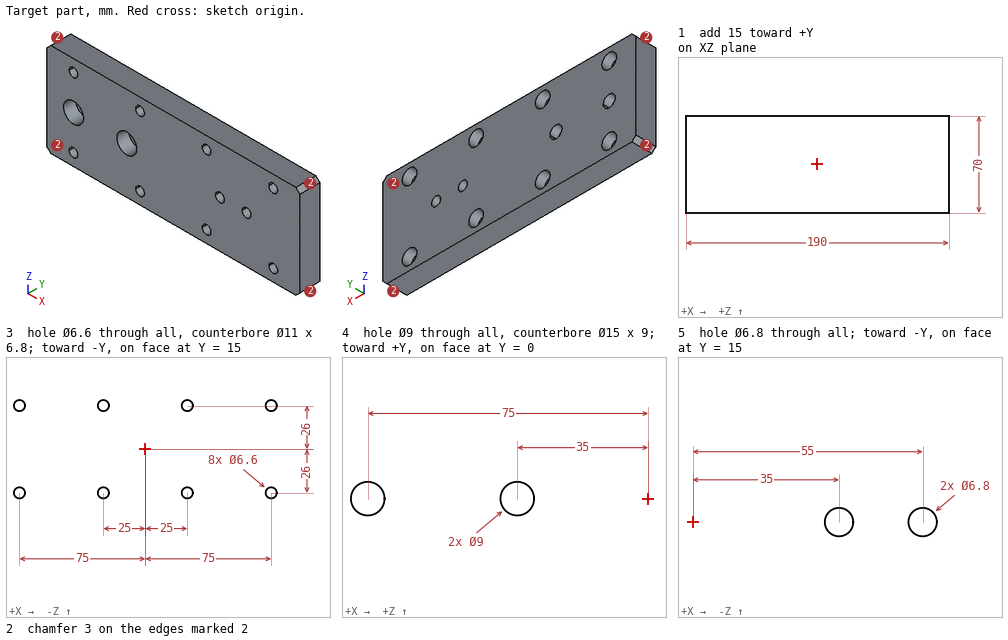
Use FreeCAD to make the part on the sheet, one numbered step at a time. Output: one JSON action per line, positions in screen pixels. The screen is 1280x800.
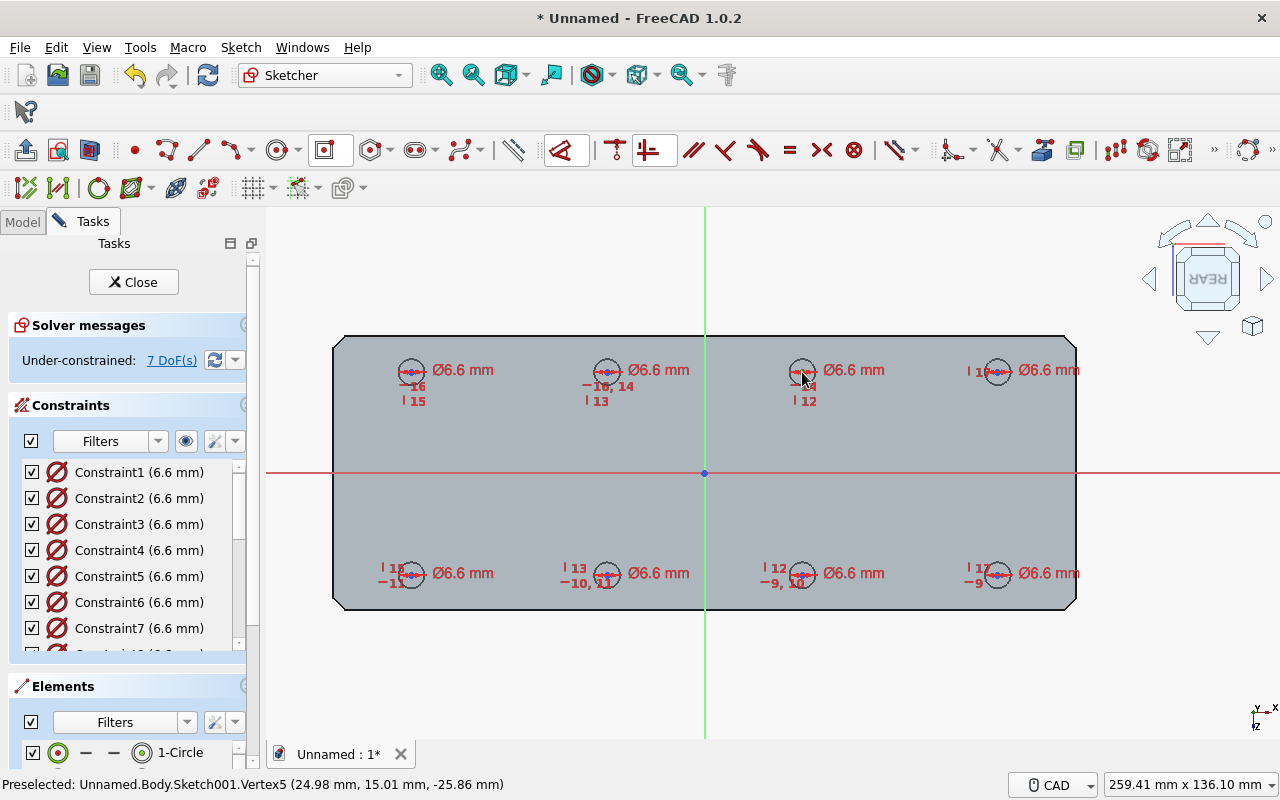
{"action": "left_click", "coordinate": [998, 372]}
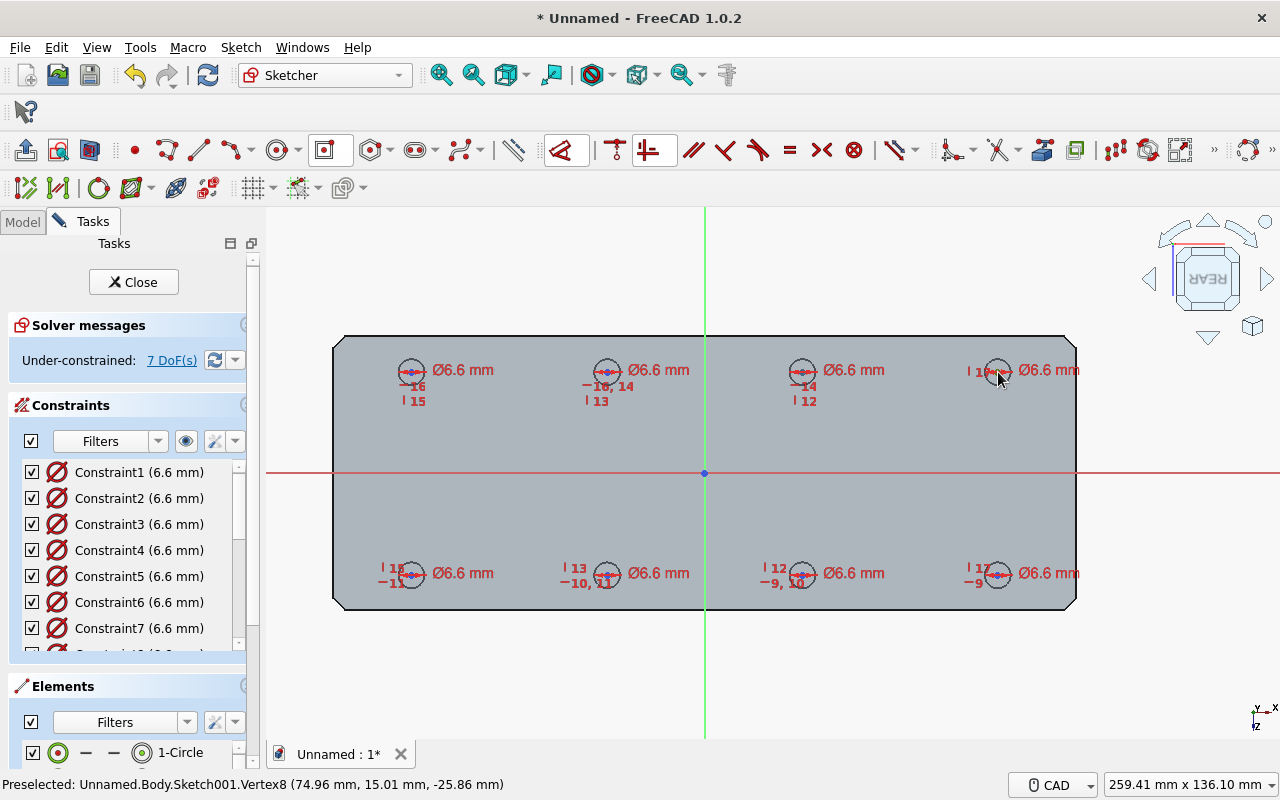
{"action": "key", "text": "h"}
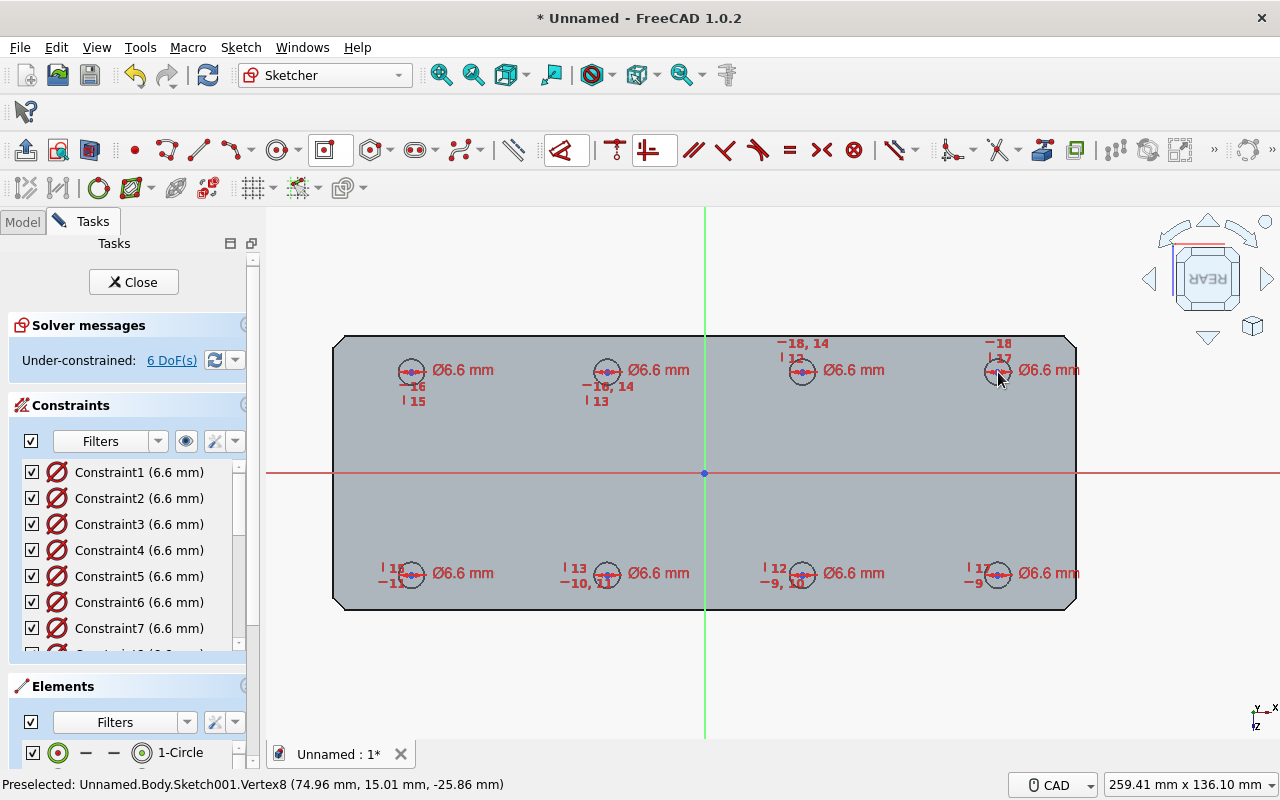
{"action": "key", "text": "d"}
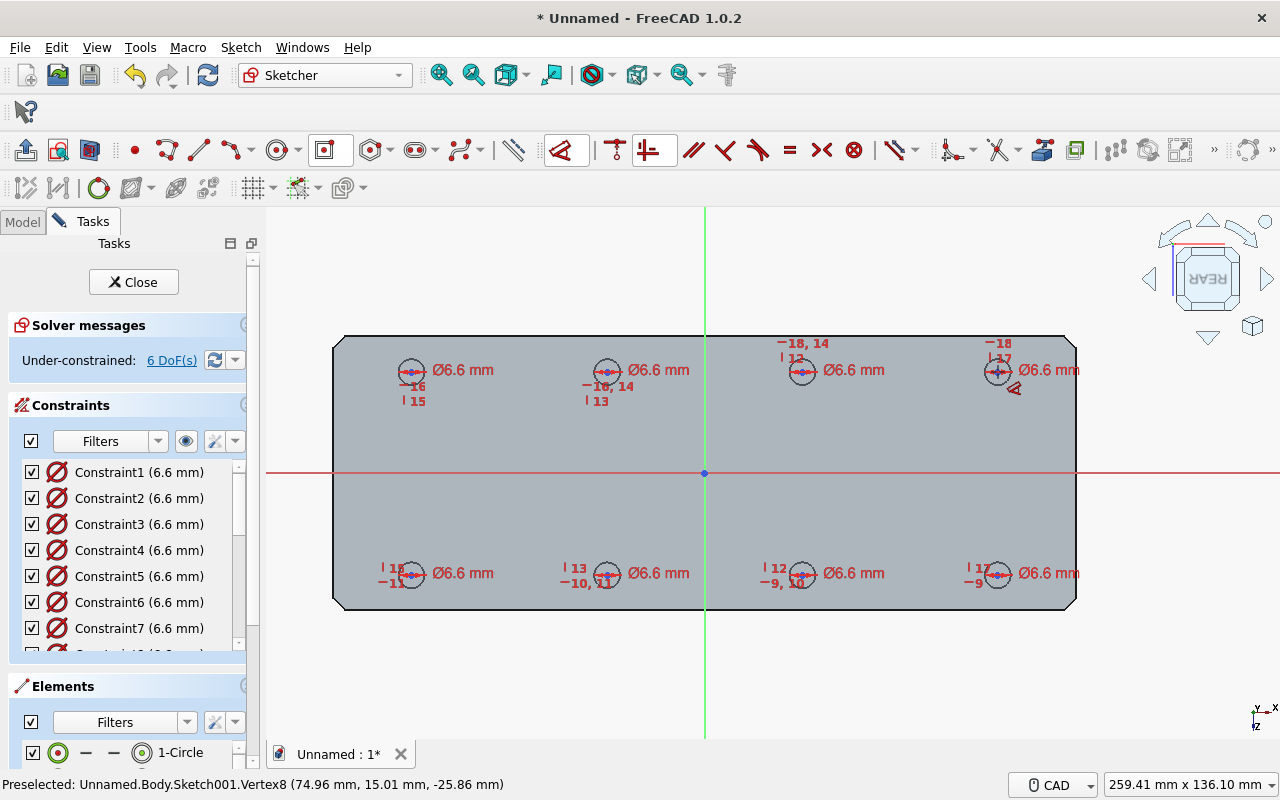
{"action": "left_click", "coordinate": [998, 575]}
{"action": "left_click", "coordinate": [851, 609]}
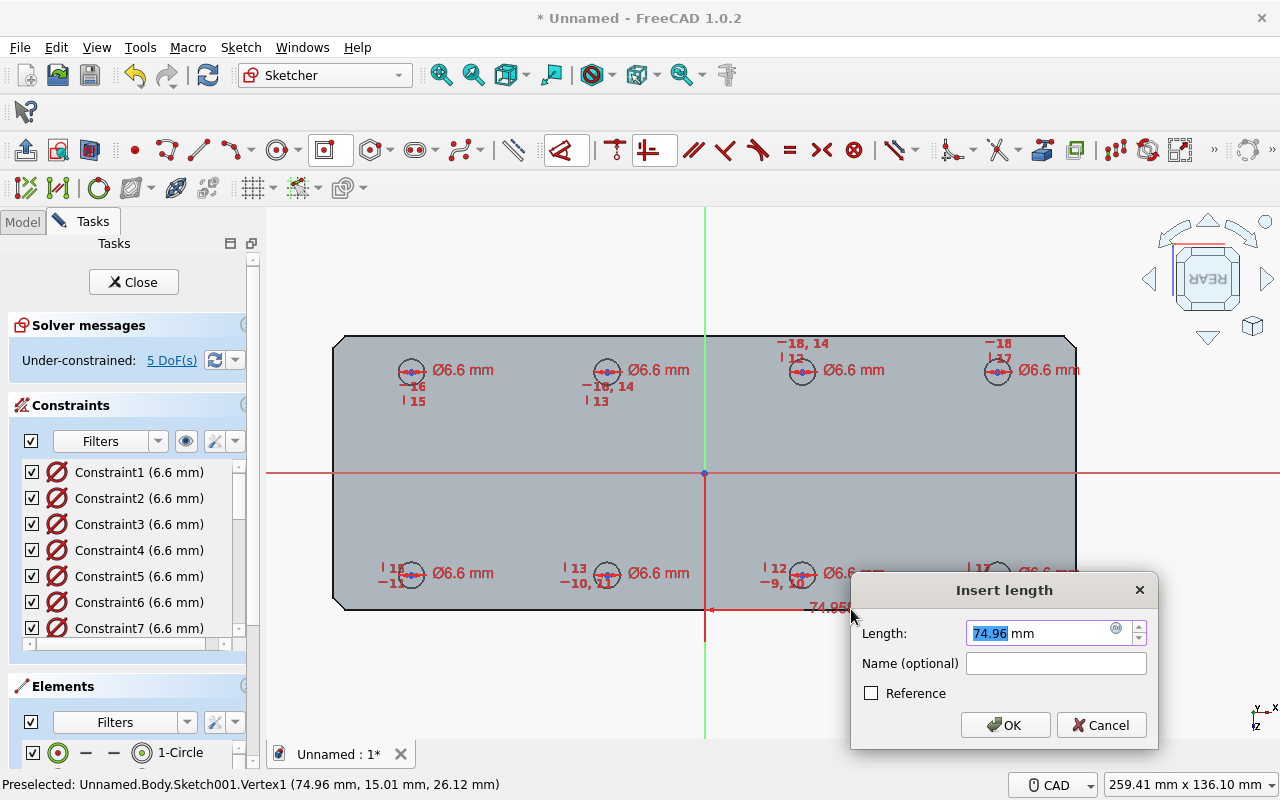
{"action": "type", "text": "75"}
{"action": "key", "text": "Return"}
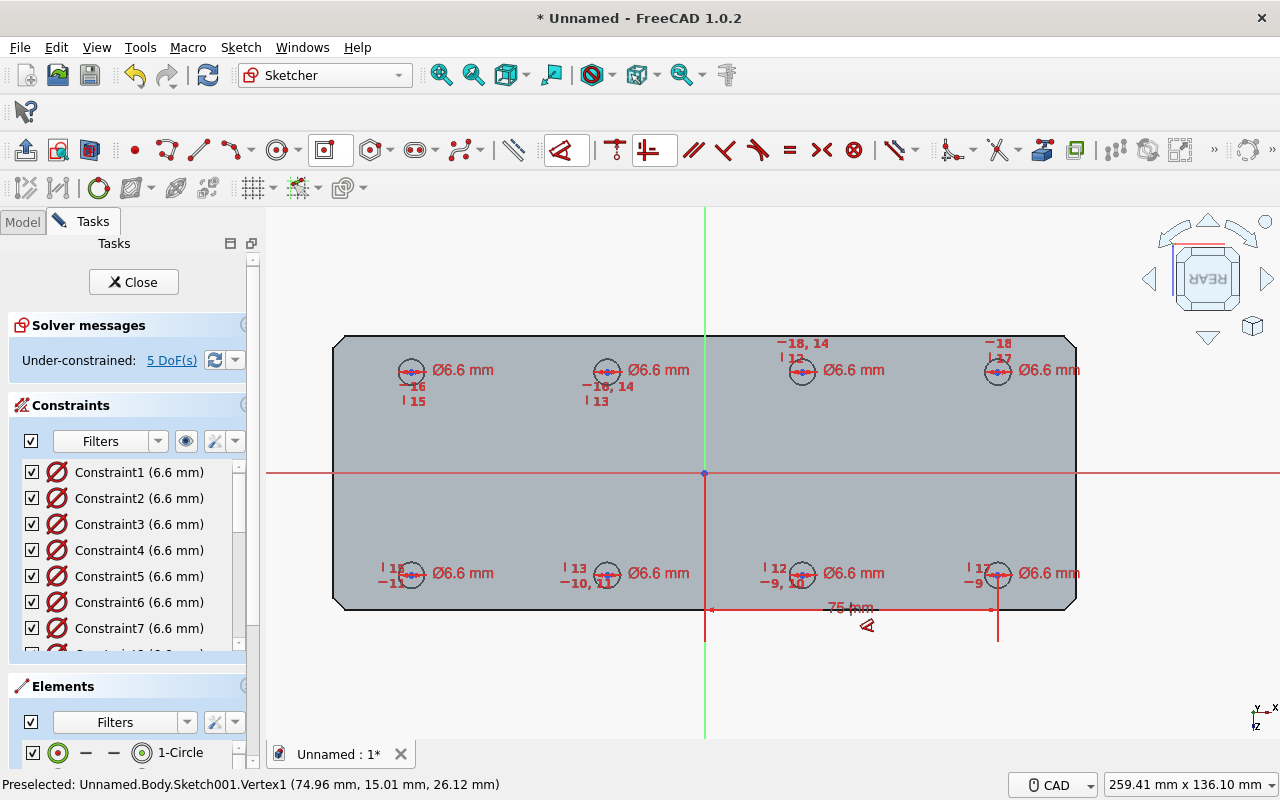
{"action": "left_click", "coordinate": [998, 575]}
{"action": "left_click", "coordinate": [1032, 524]}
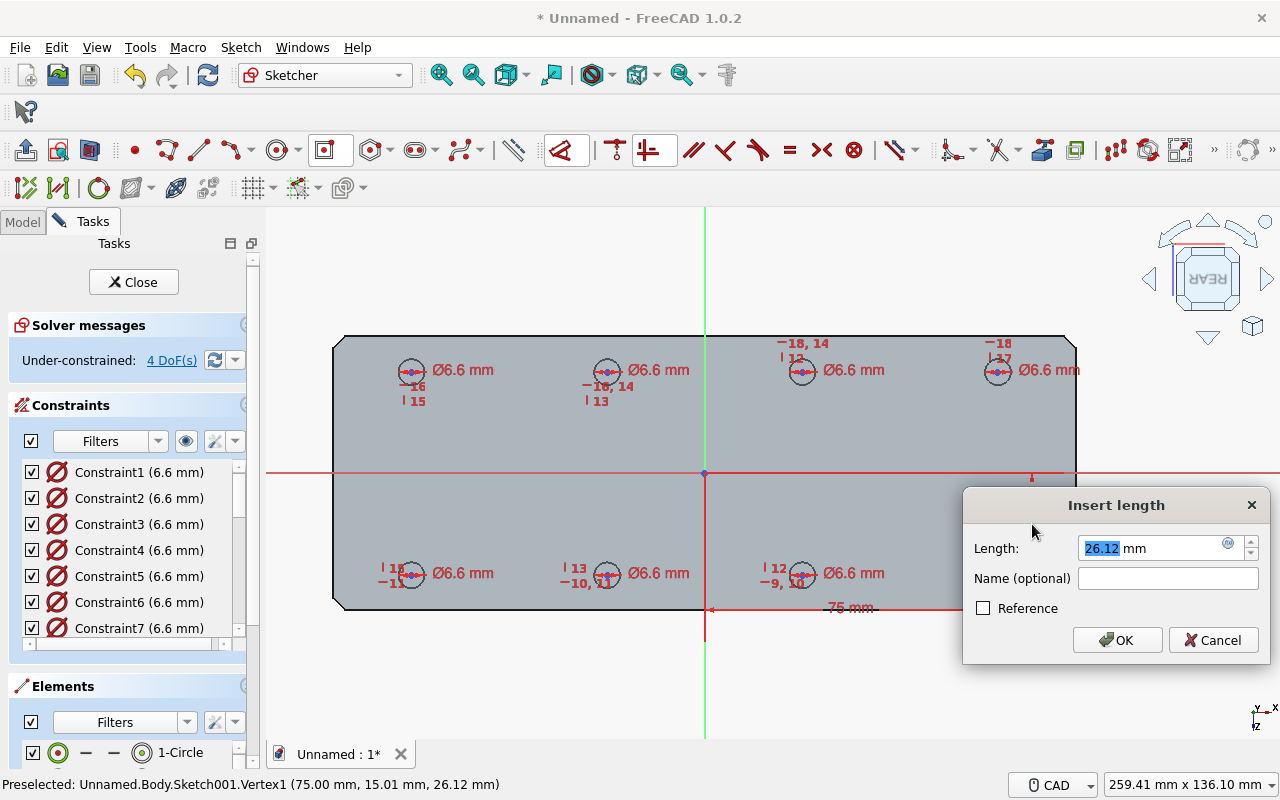
{"action": "type", "text": "26"}
{"action": "key", "text": "Return"}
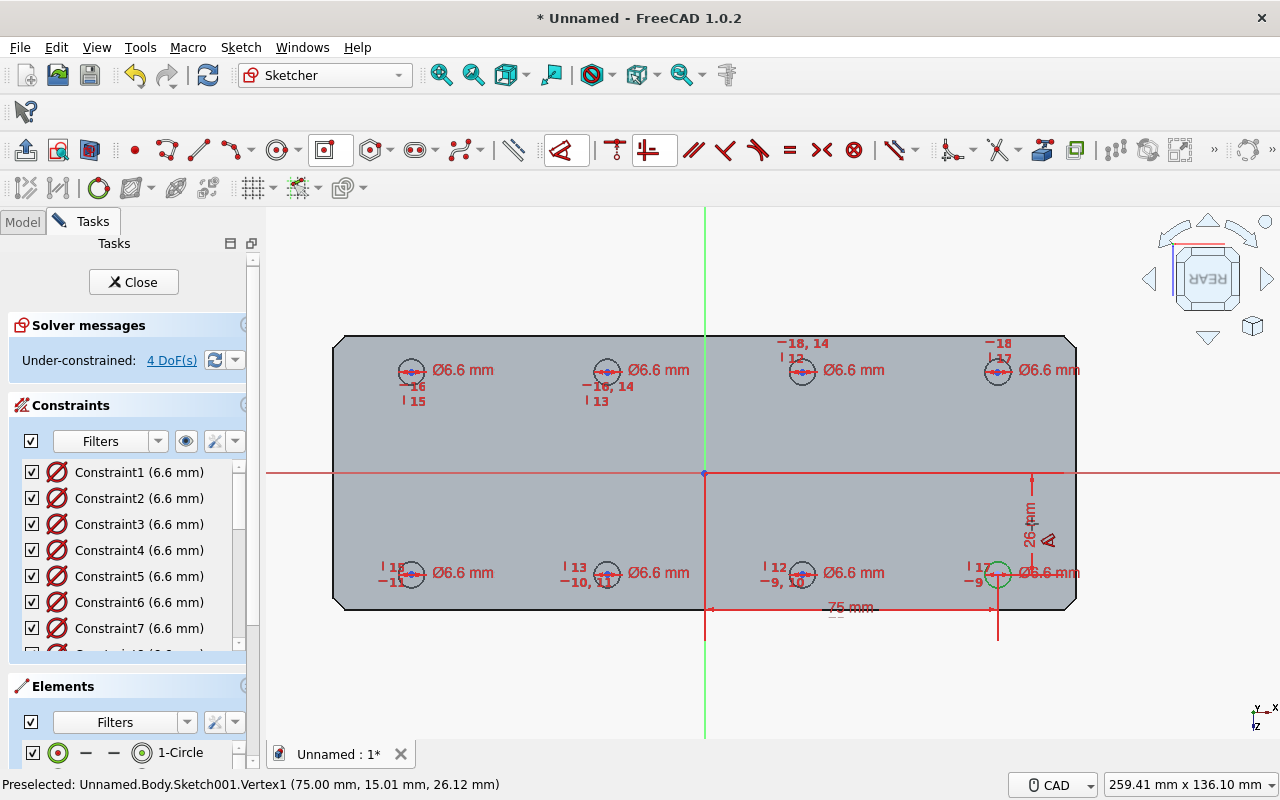
{"action": "left_click", "coordinate": [802, 575]}
{"action": "left_click", "coordinate": [754, 609]}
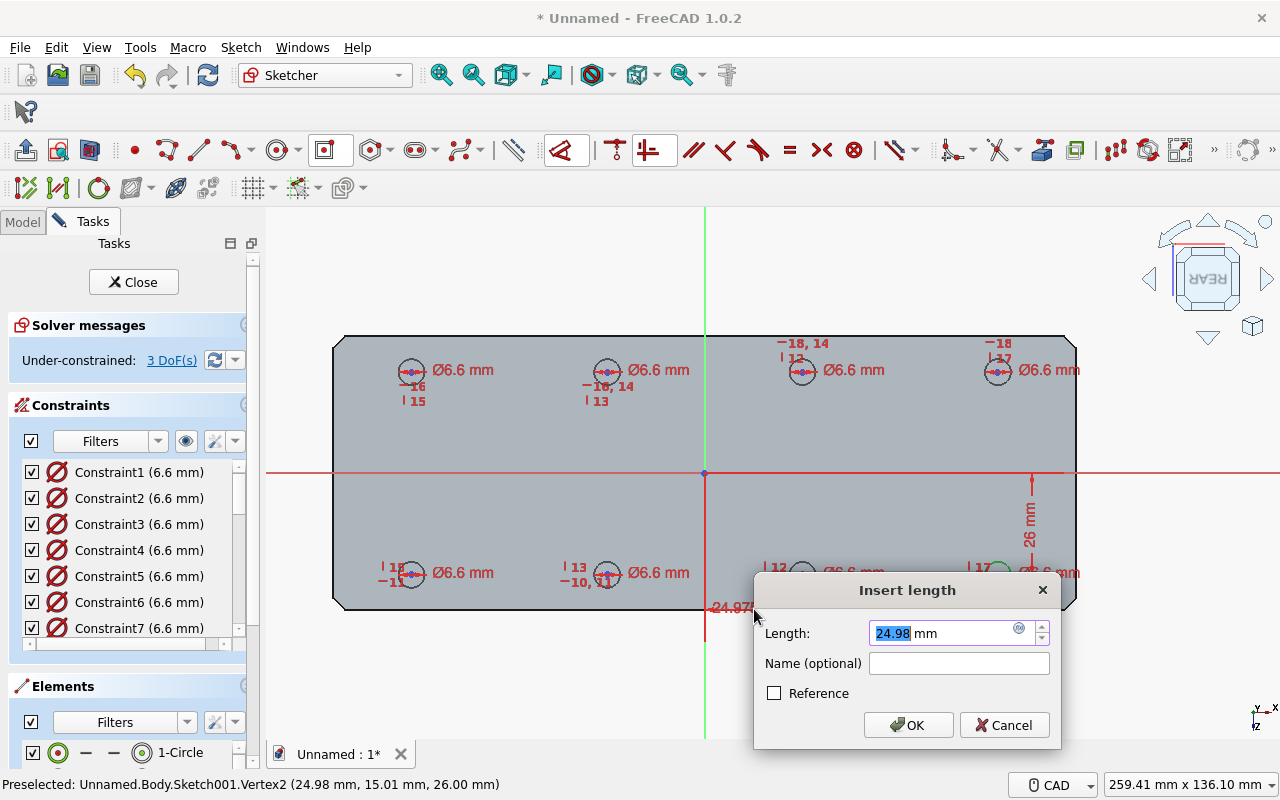
{"action": "type", "text": "25"}
{"action": "key", "text": "Return"}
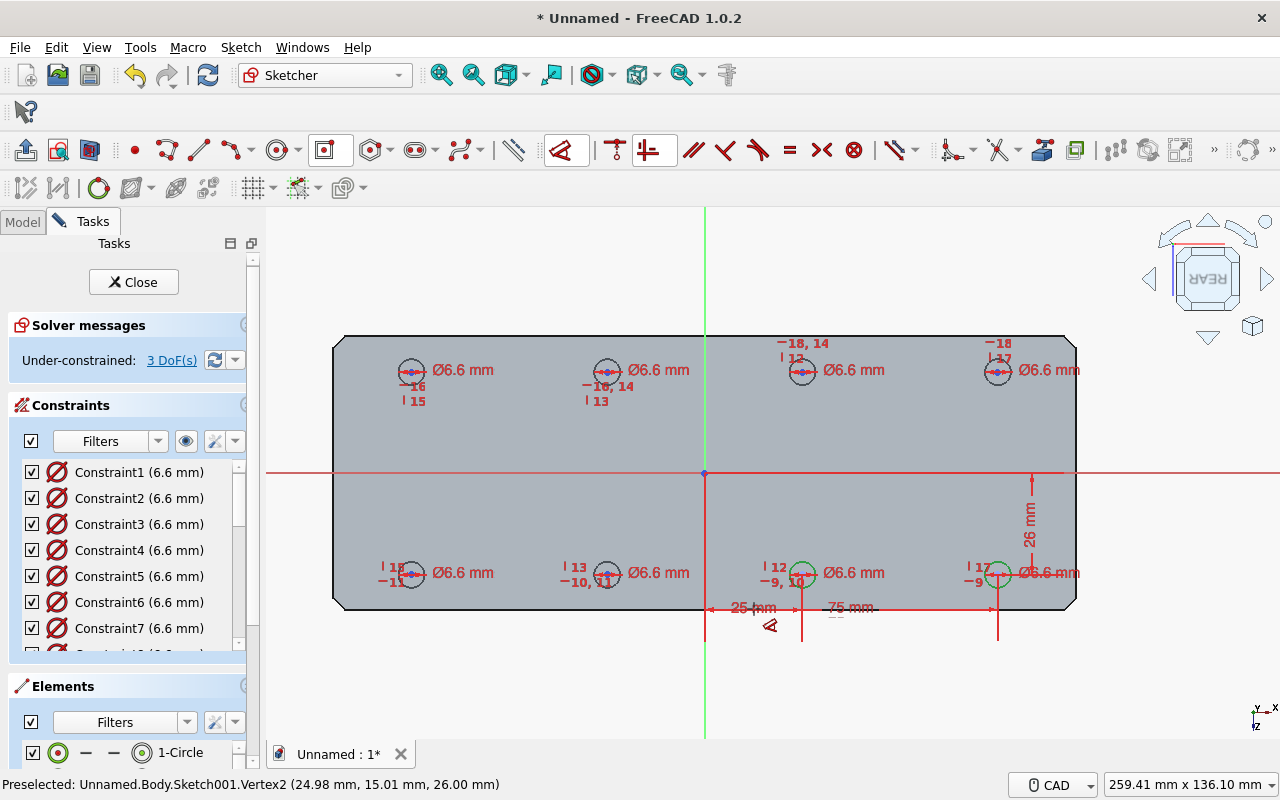
{"action": "left_click", "coordinate": [607, 575]}
{"action": "left_click", "coordinate": [656, 609]}